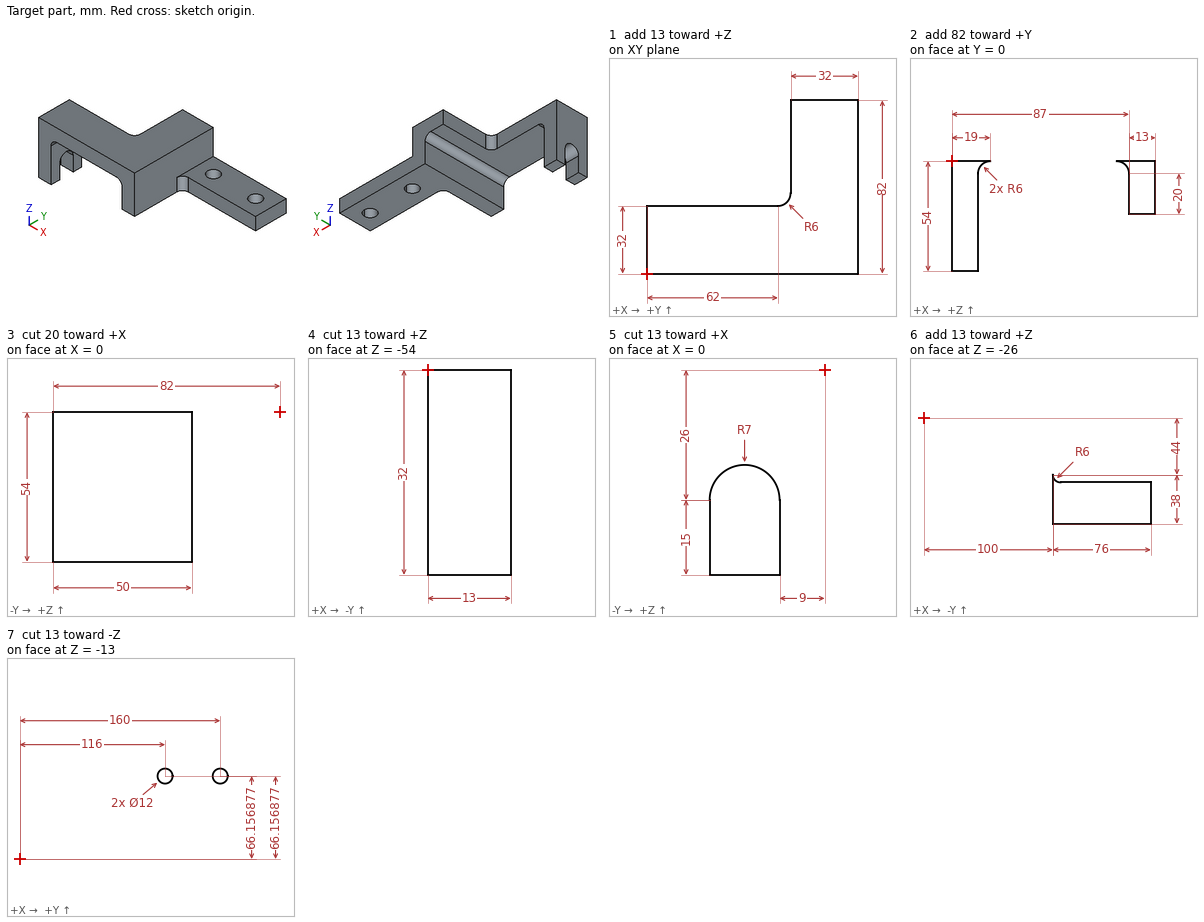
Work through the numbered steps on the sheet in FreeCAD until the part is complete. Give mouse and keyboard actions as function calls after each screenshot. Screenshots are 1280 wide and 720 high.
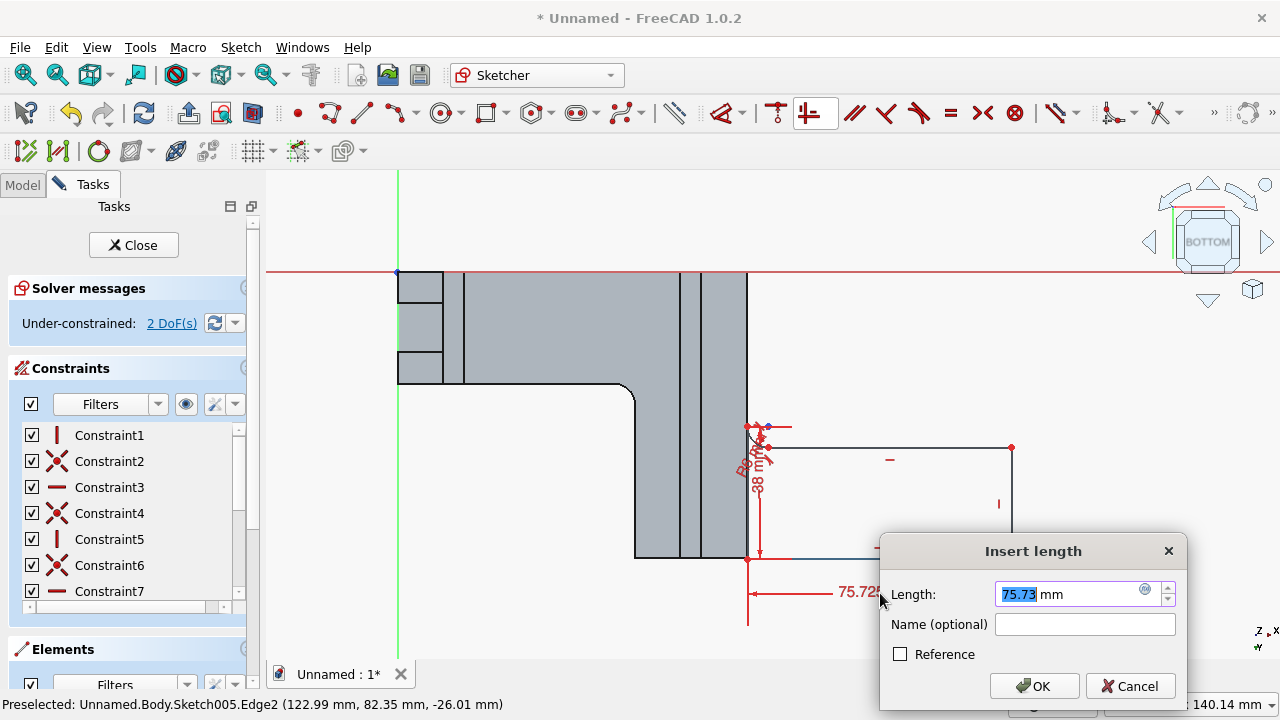
text(76)
key(Return)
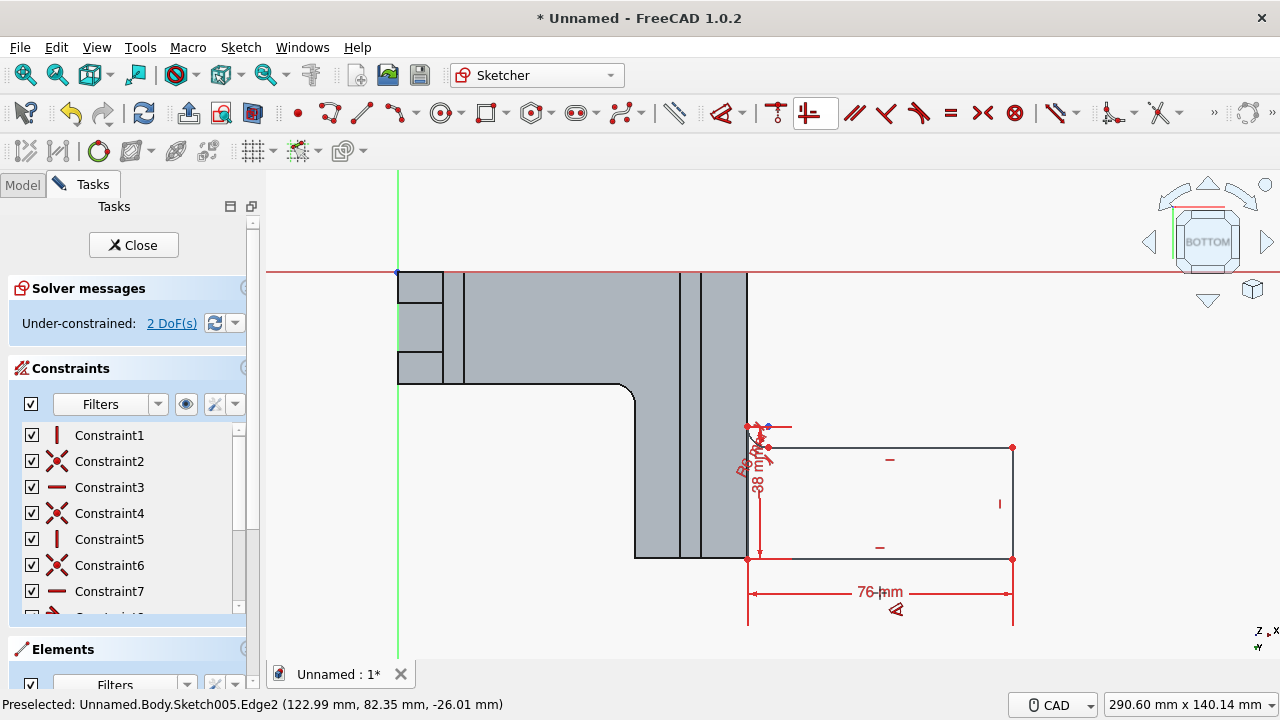
click(748, 427)
click(364, 349)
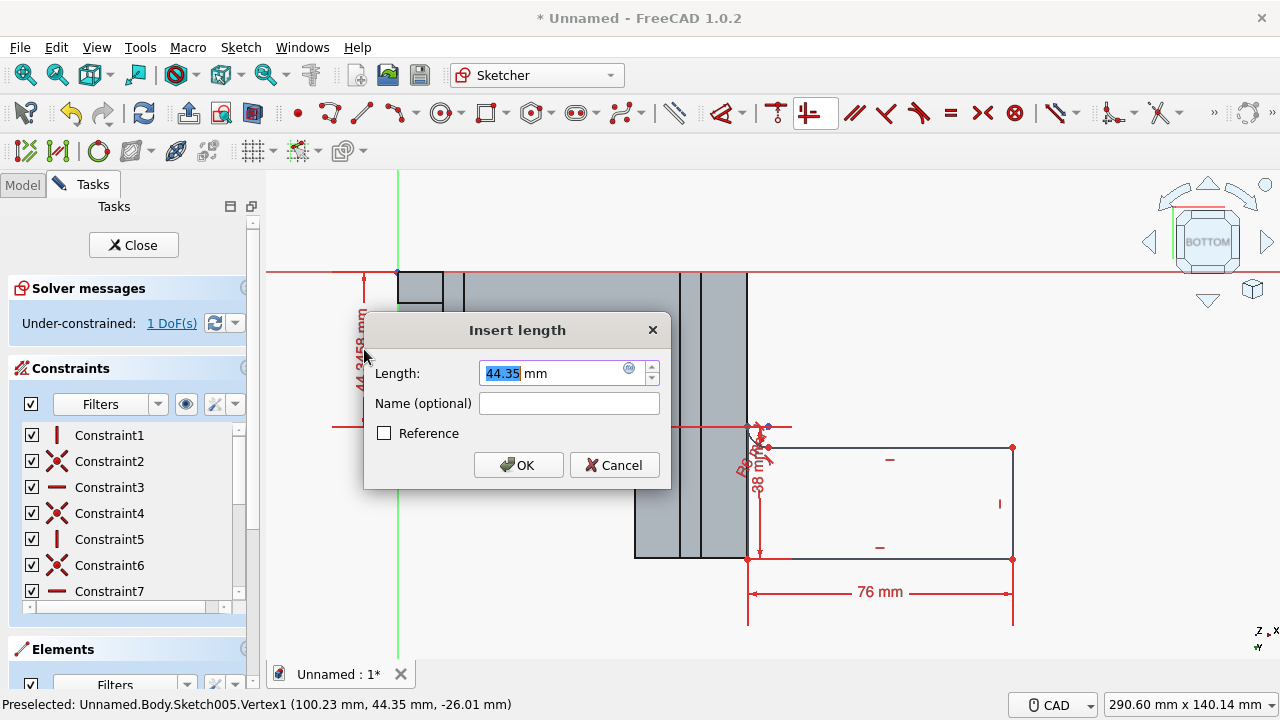
text(44)
key(Return)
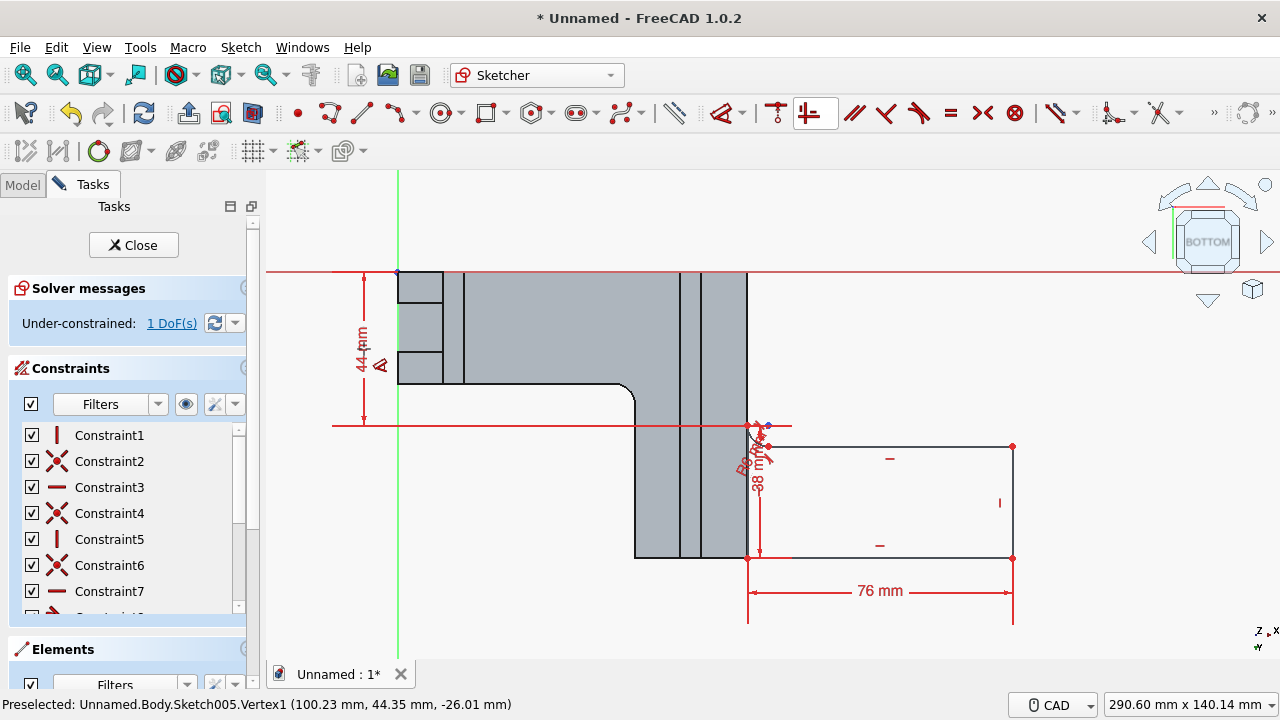
click(748, 426)
click(573, 238)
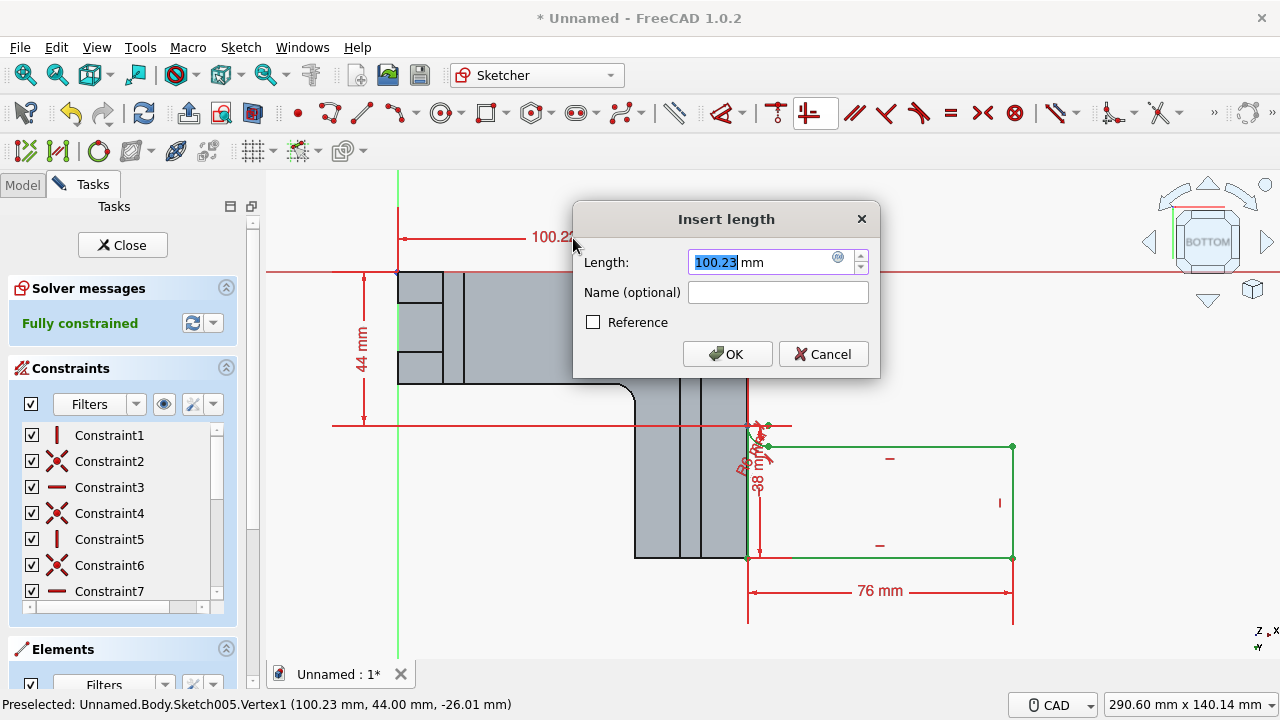
text(100)
key(Return)
key(Escape)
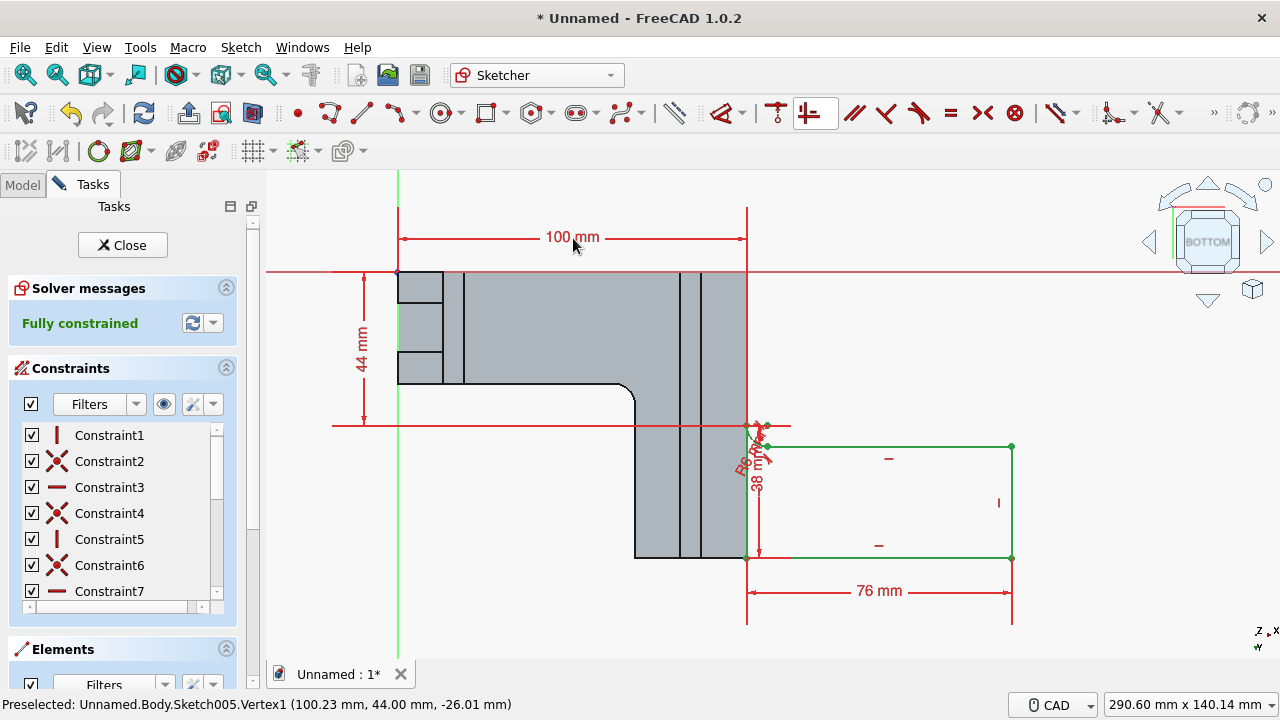
click(123, 245)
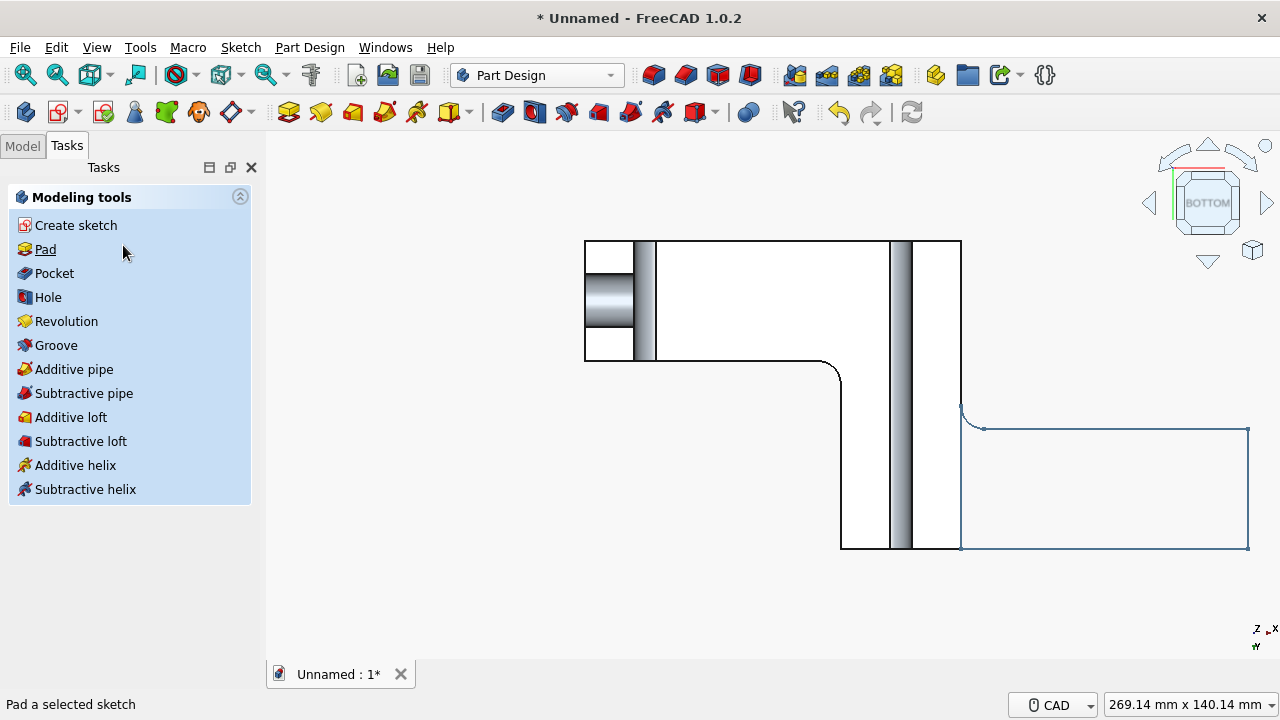
click(290, 112)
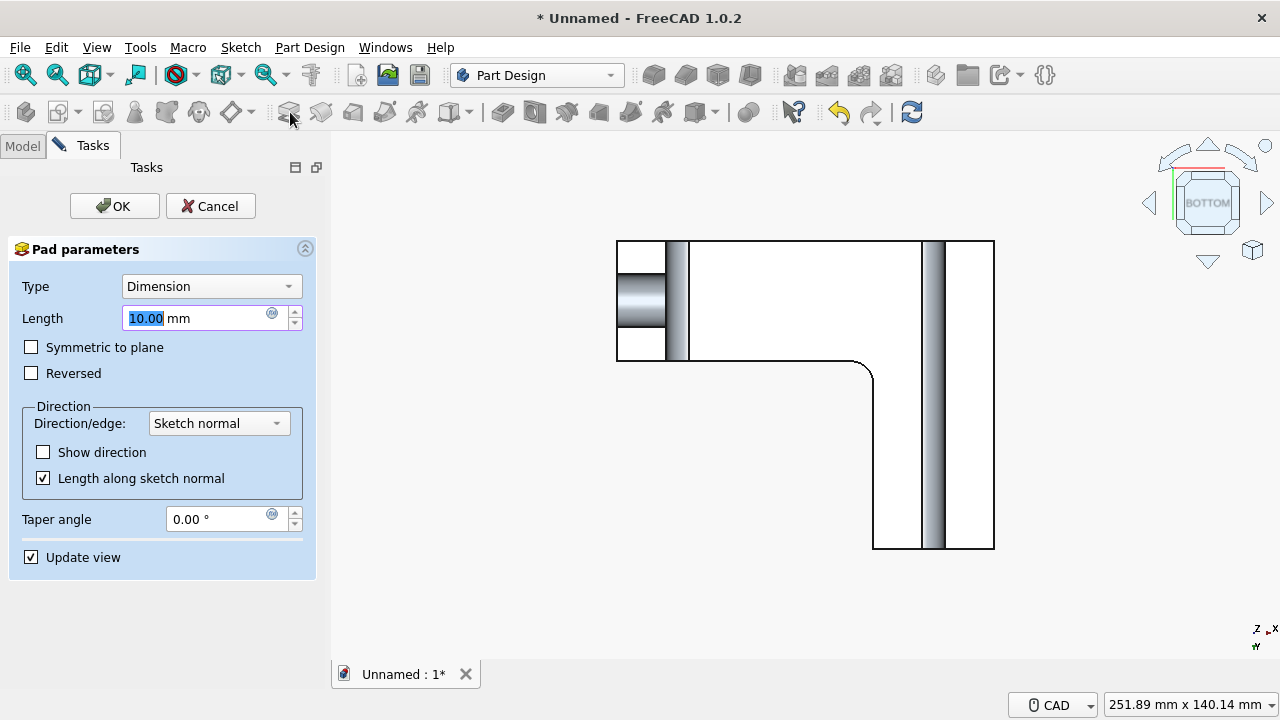
text(13)
key(Tab)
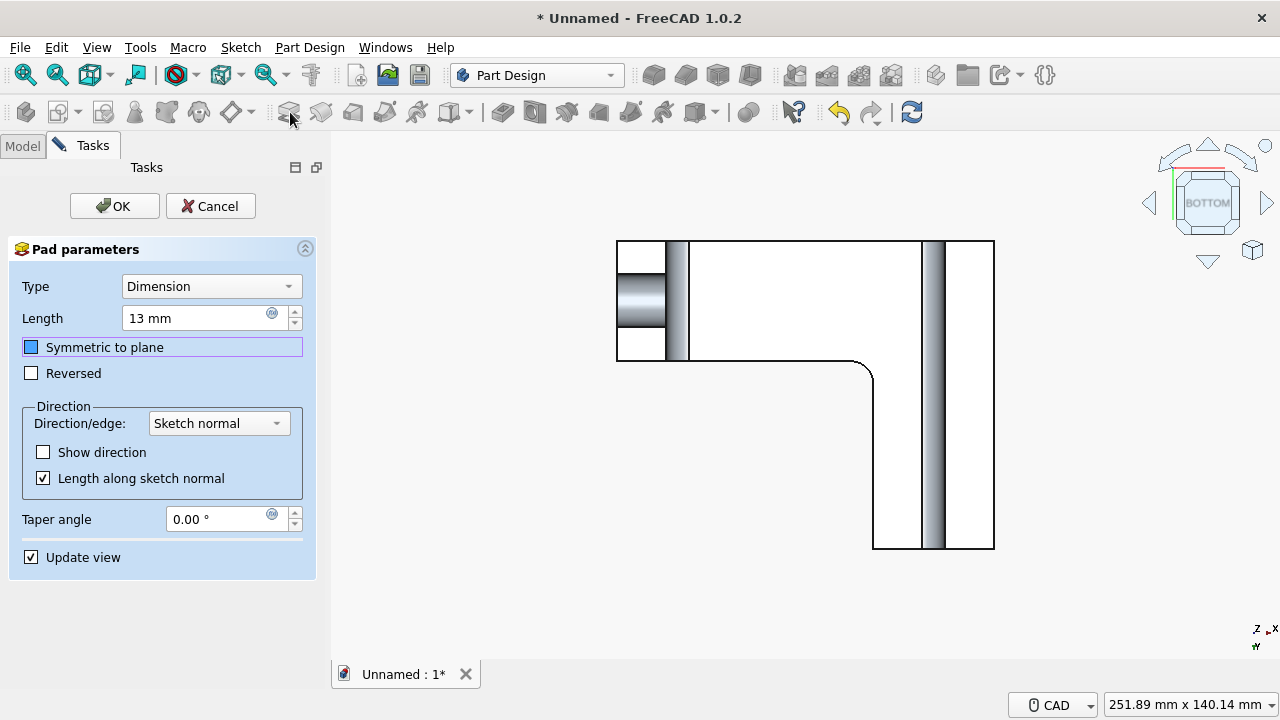
click(30, 373)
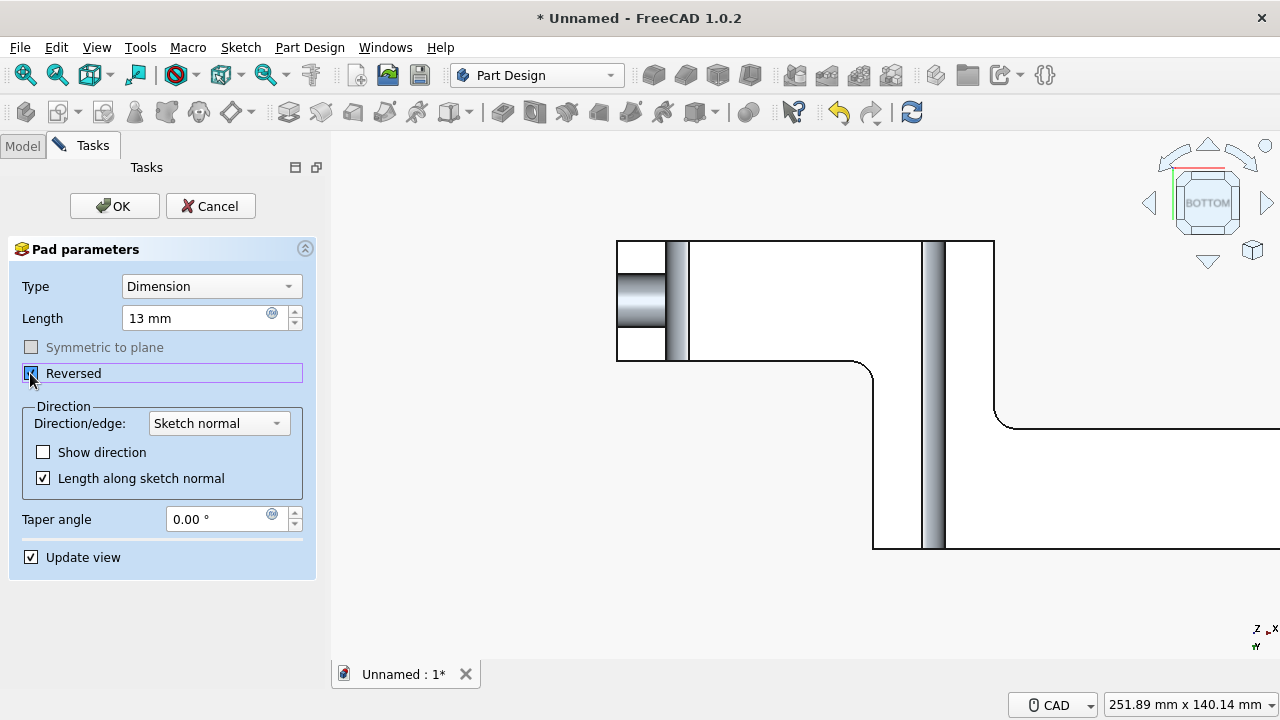
click(115, 206)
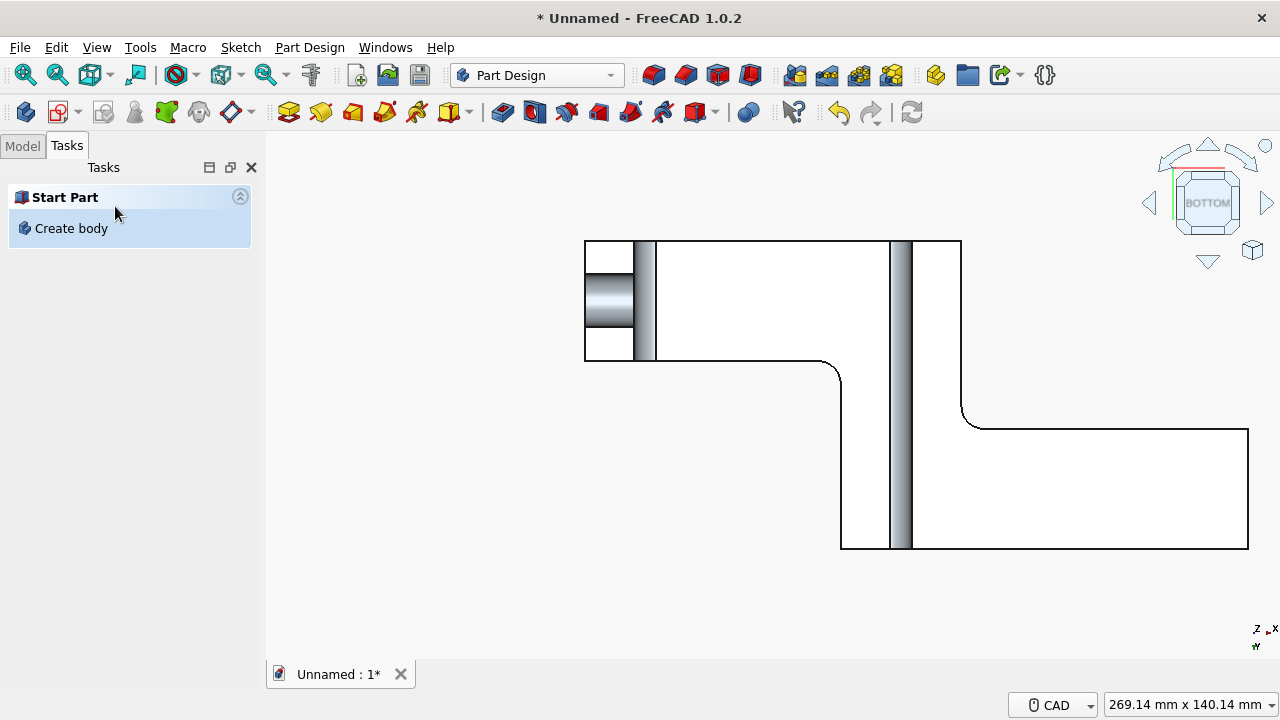
key(0)